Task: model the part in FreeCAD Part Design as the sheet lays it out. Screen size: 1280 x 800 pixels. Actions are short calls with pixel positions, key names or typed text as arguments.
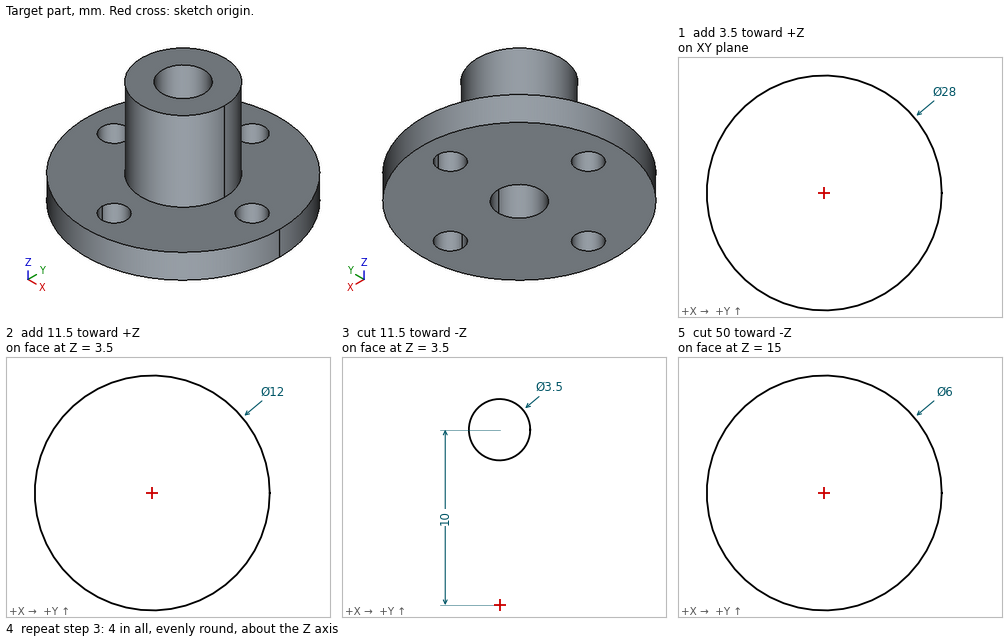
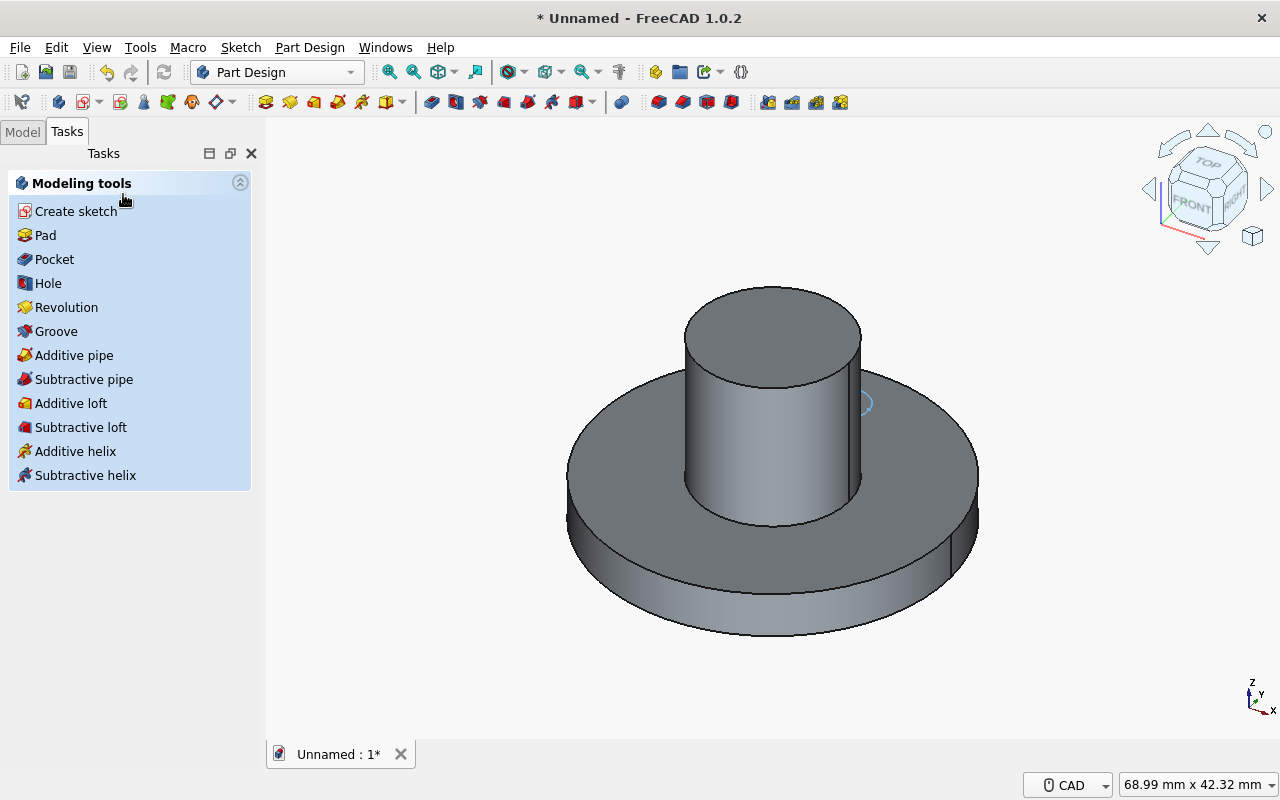
click(432, 102)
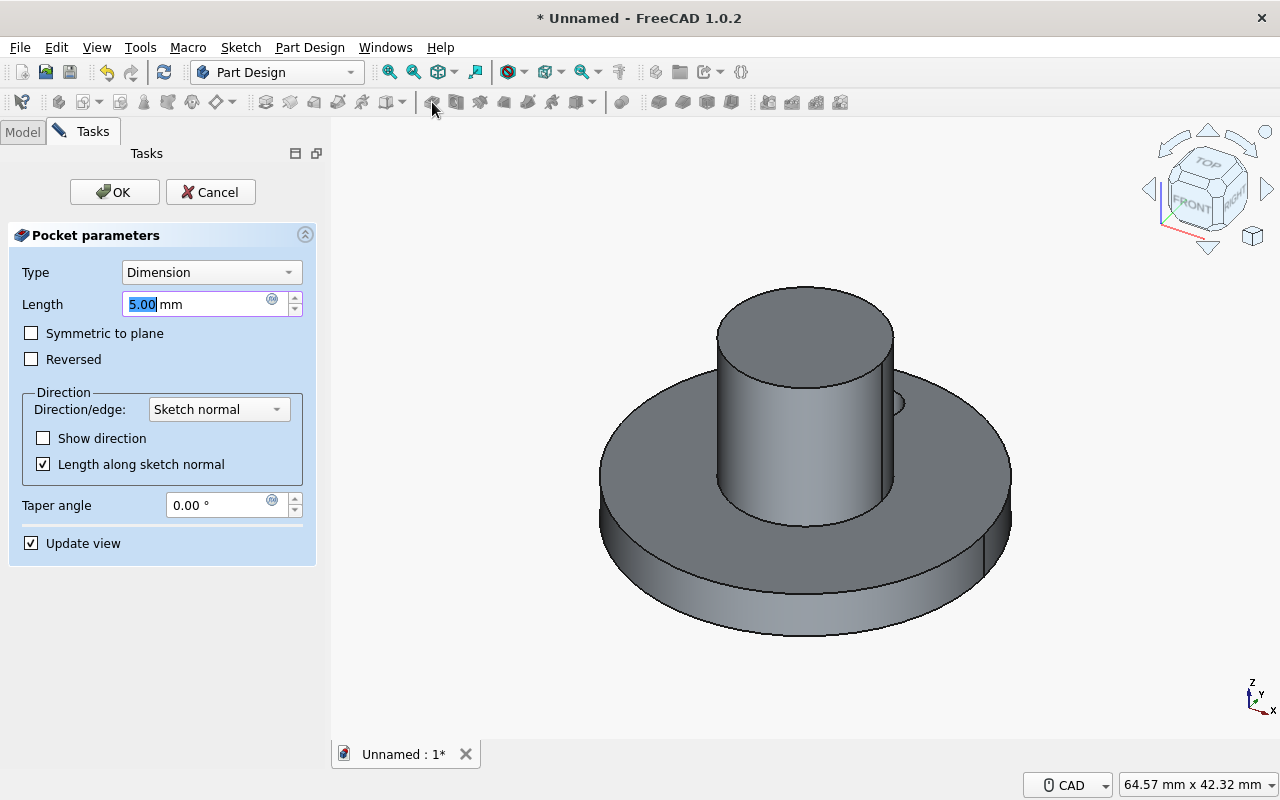
text(11.5)
key(Tab)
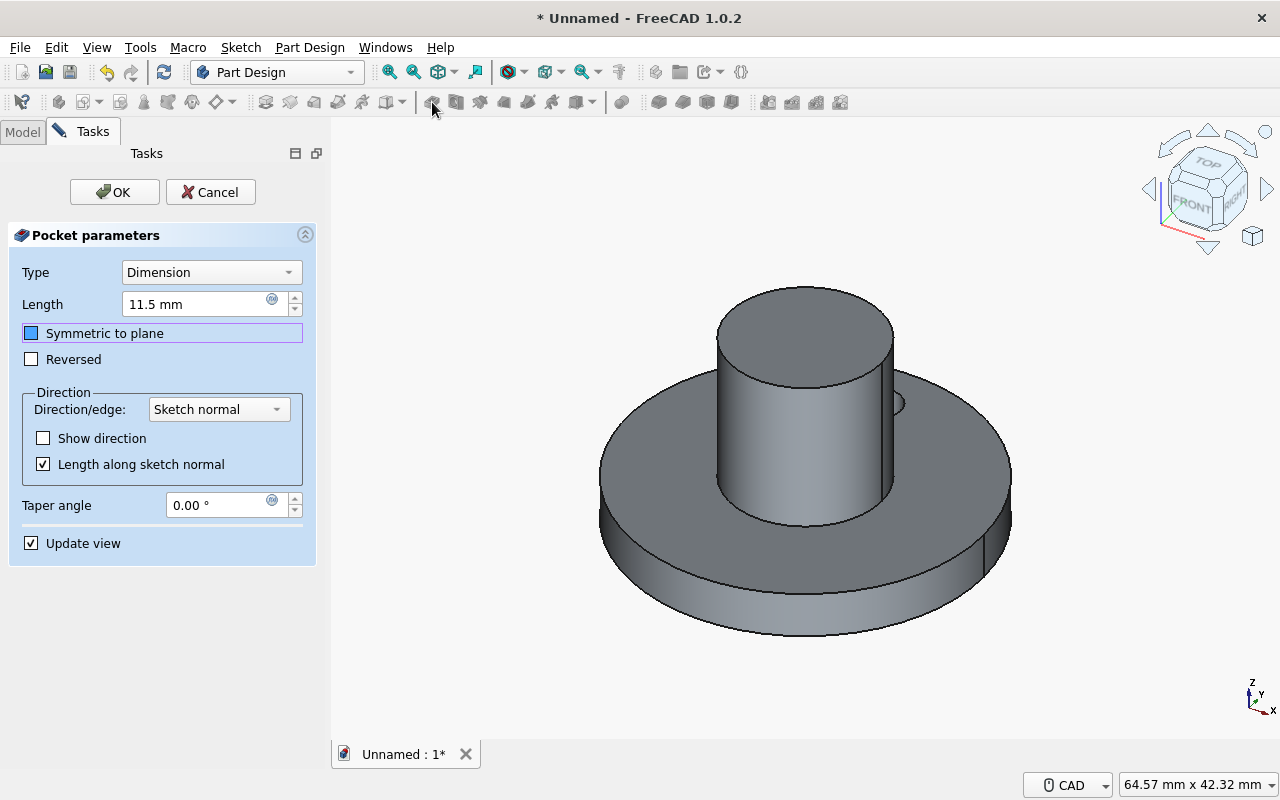
click(115, 192)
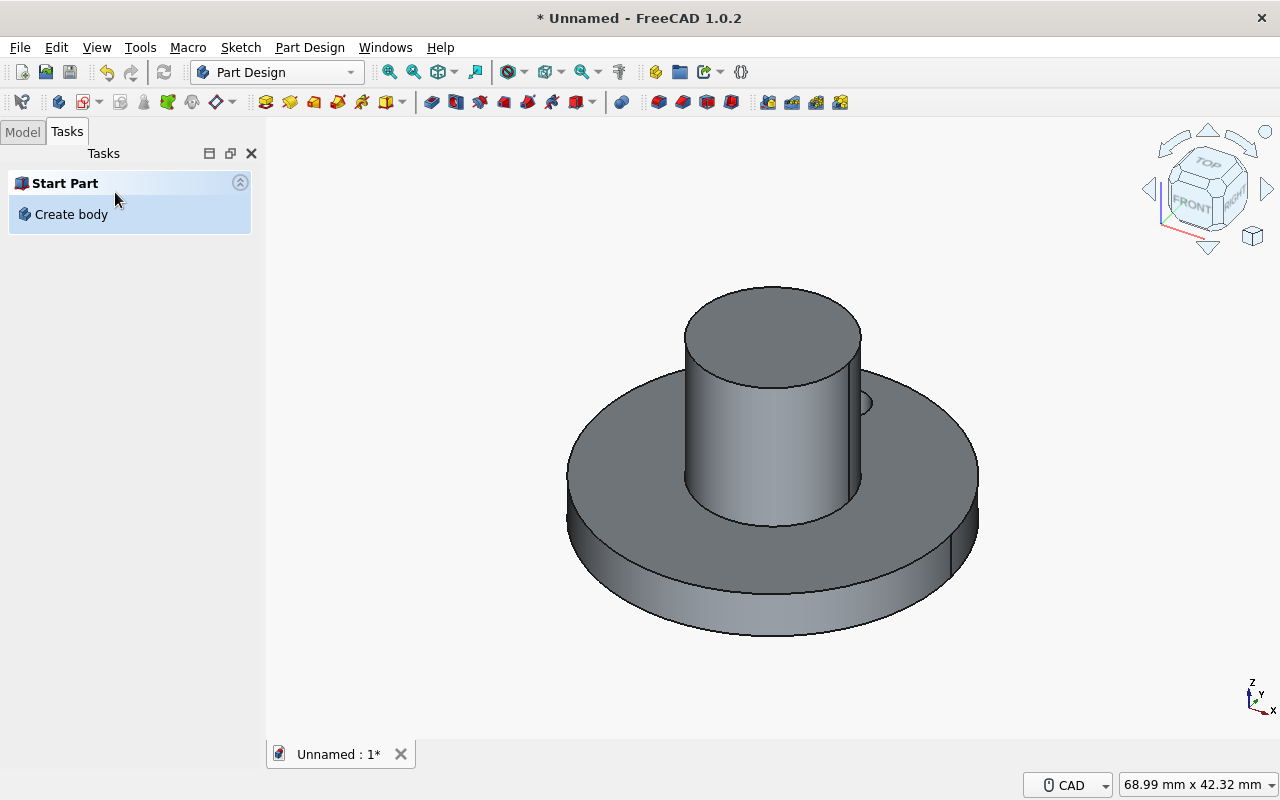
click(23, 131)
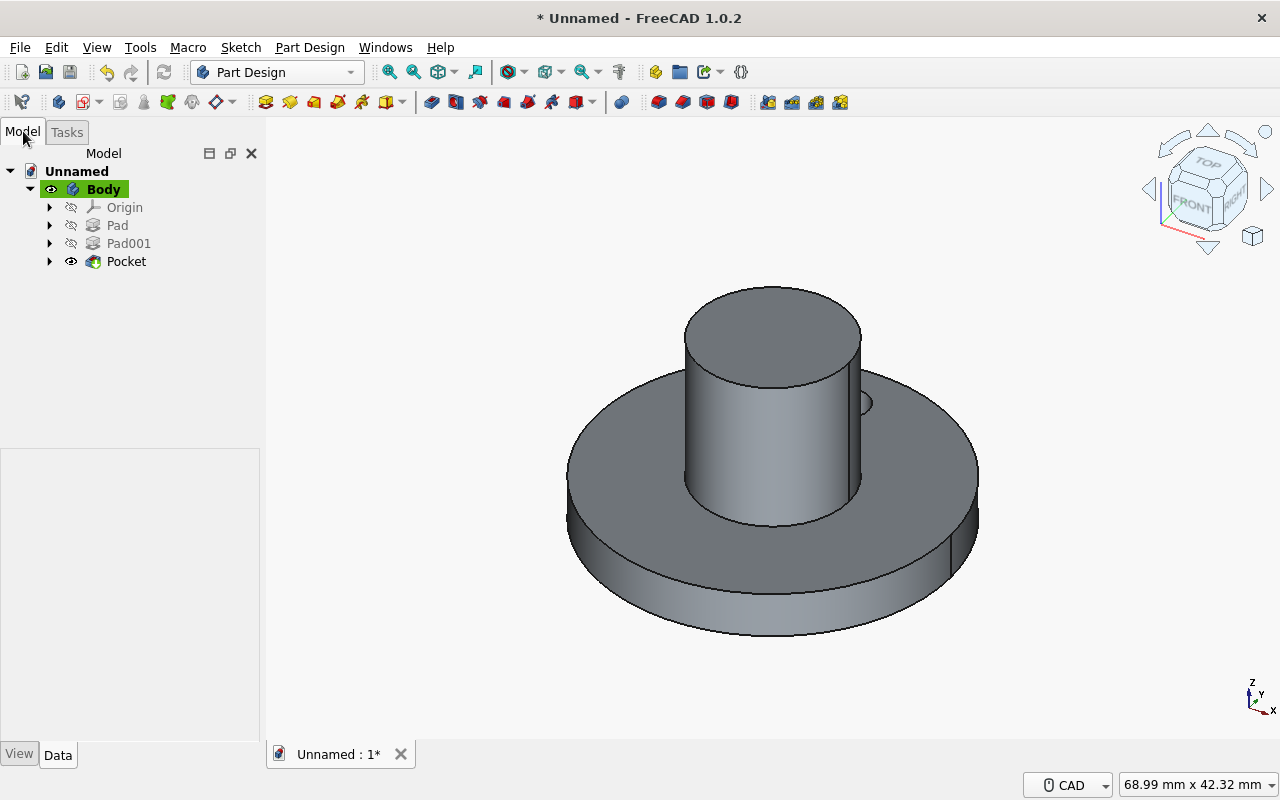
click(116, 261)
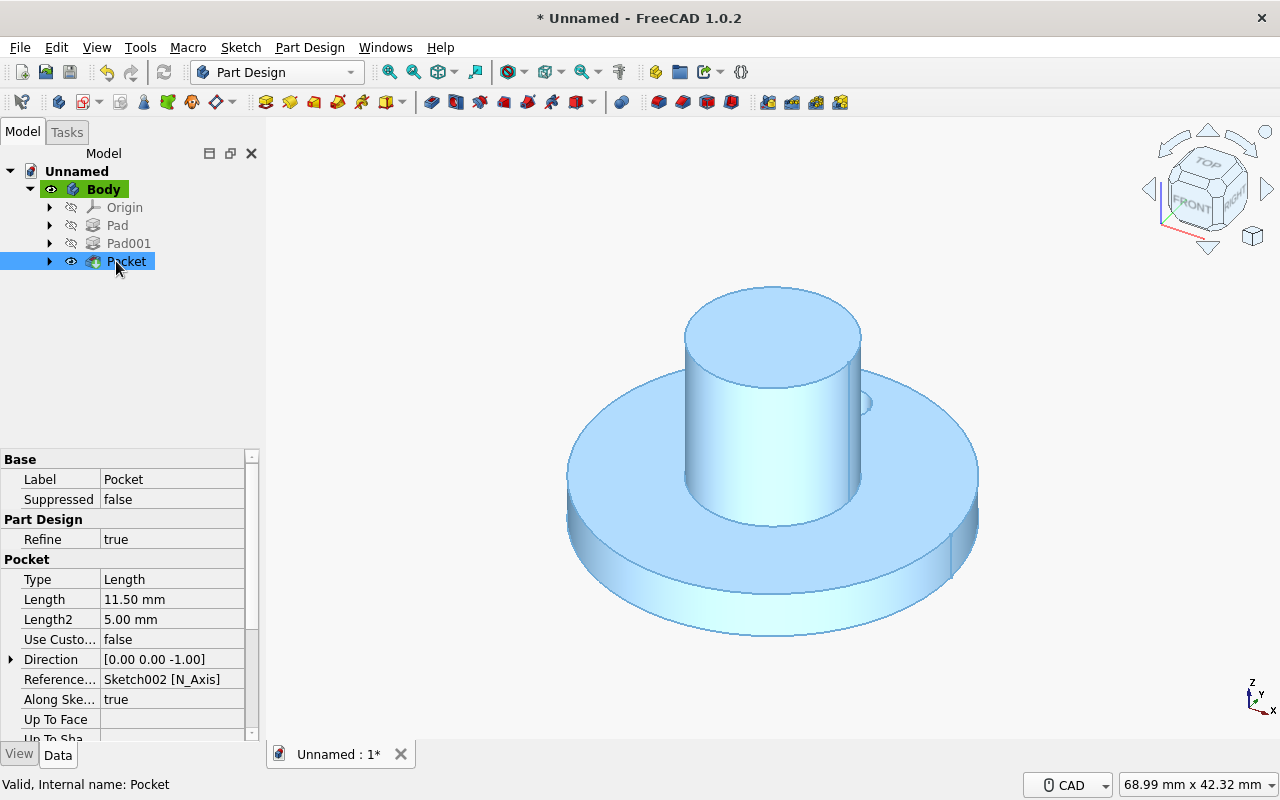
click(816, 102)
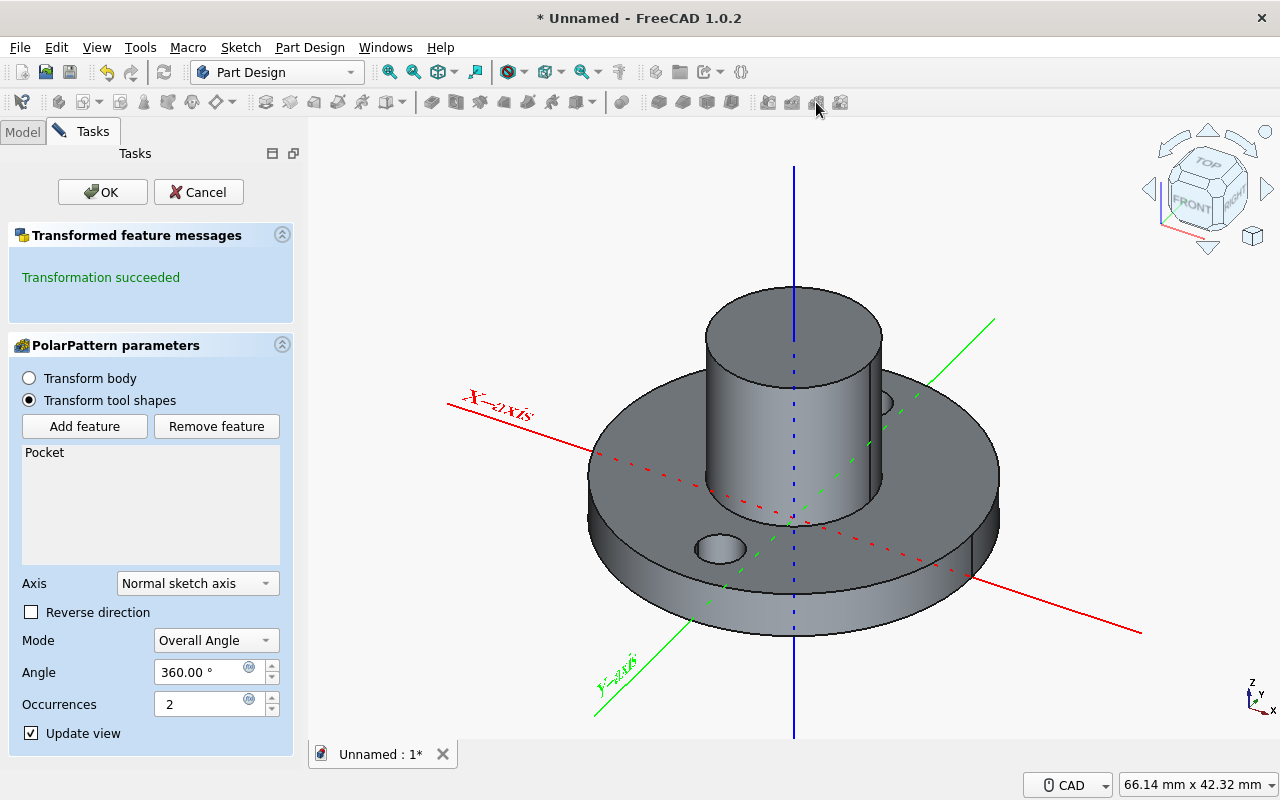
click(198, 584)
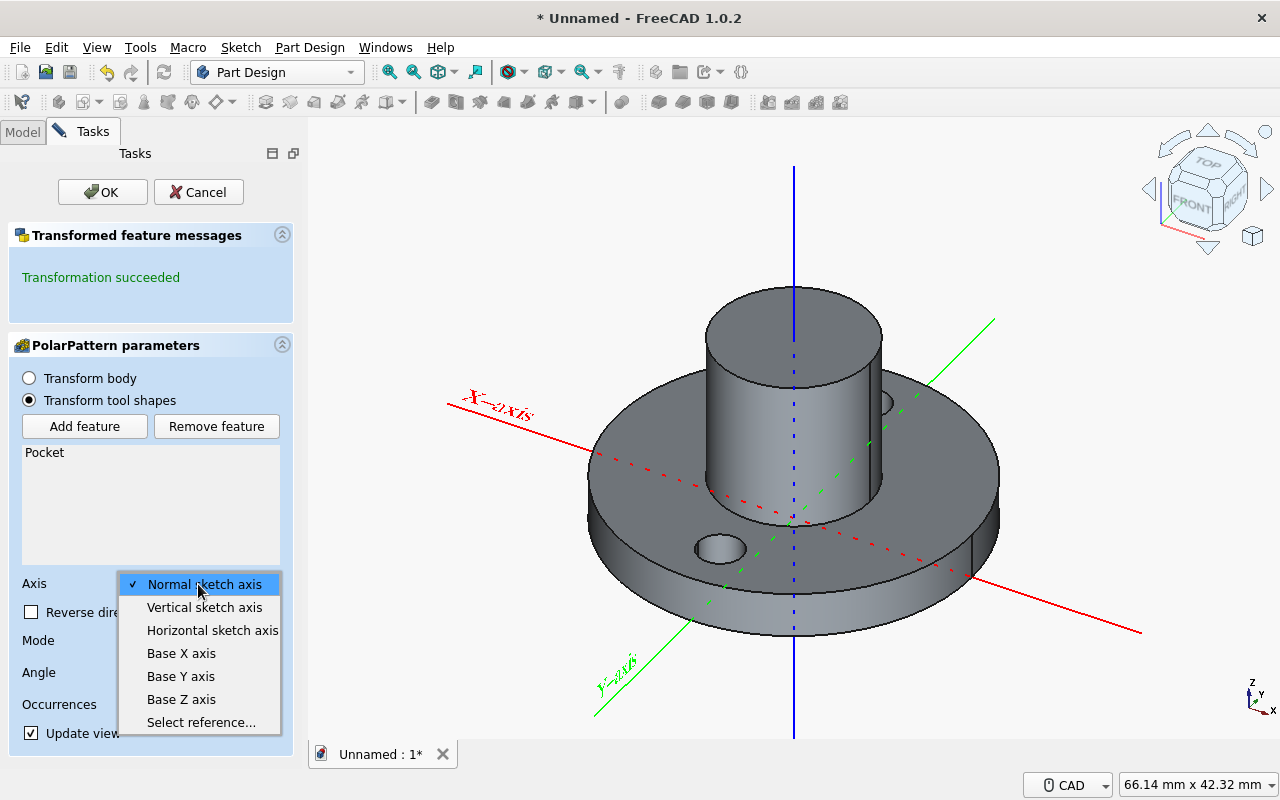
click(198, 700)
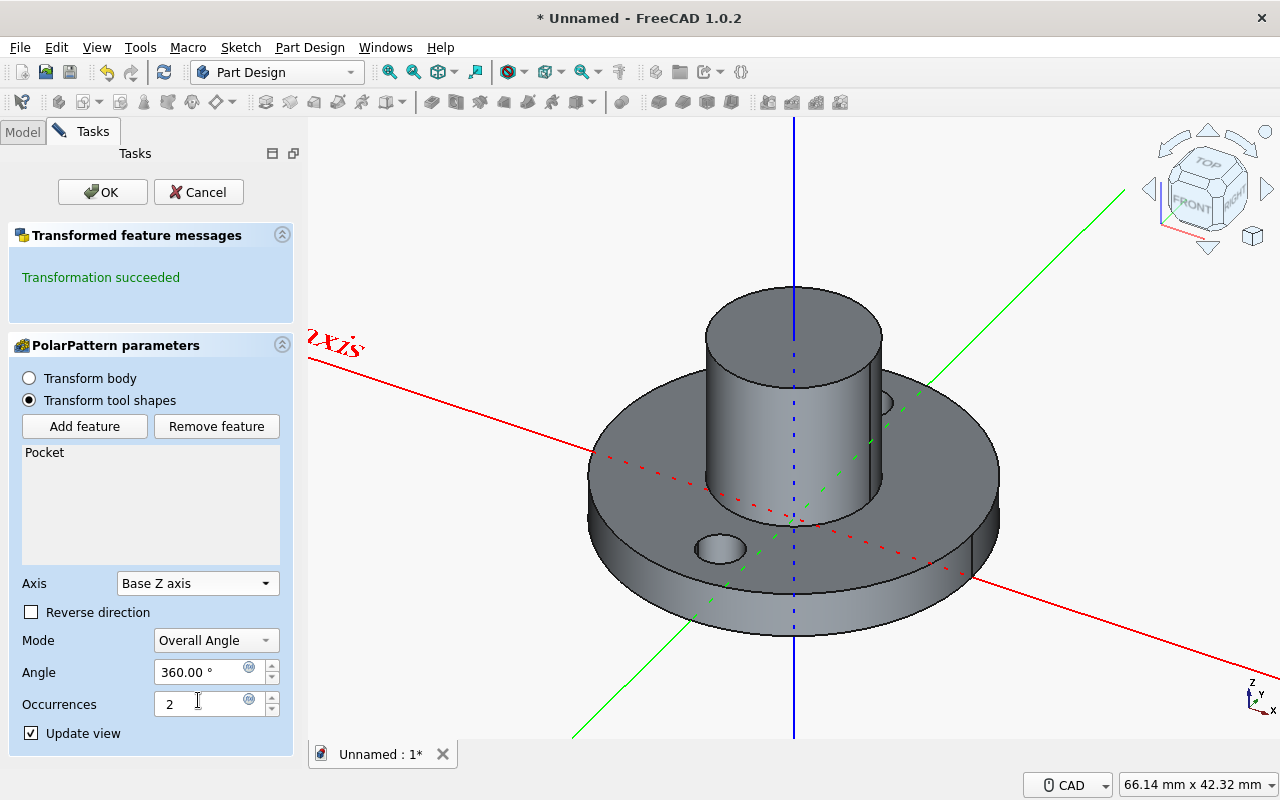
triple_click(209, 704)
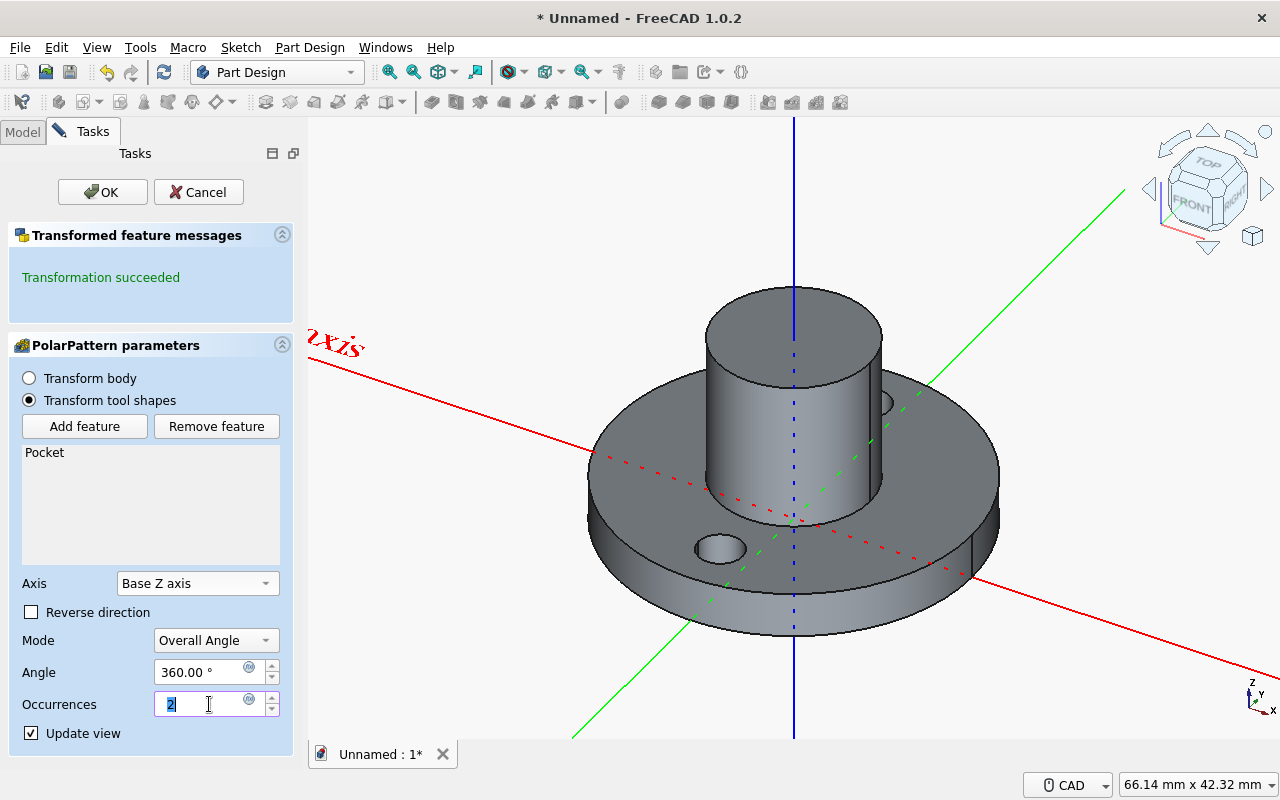
text(4)
key(Tab)